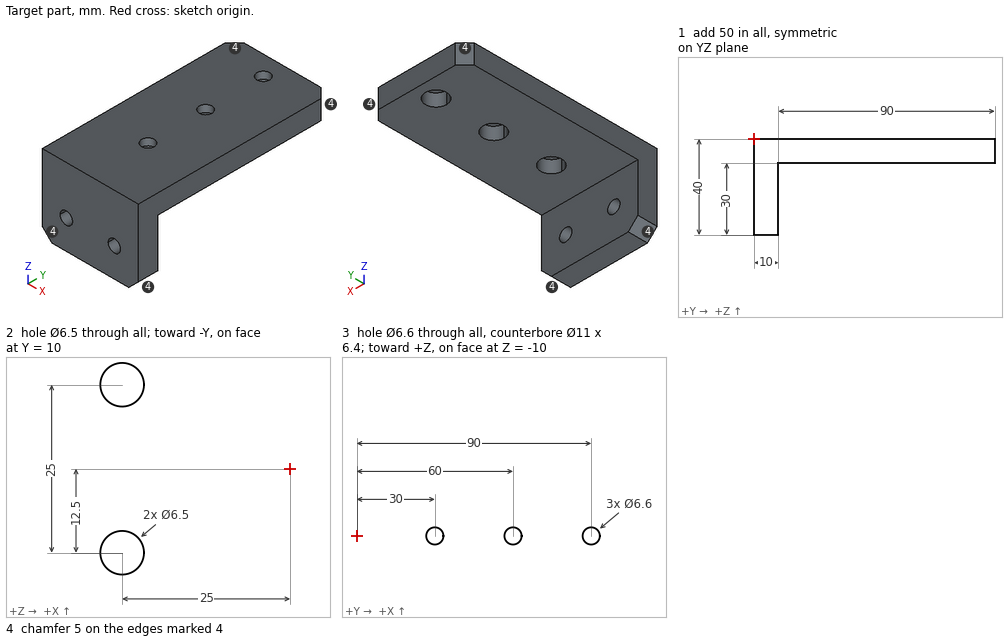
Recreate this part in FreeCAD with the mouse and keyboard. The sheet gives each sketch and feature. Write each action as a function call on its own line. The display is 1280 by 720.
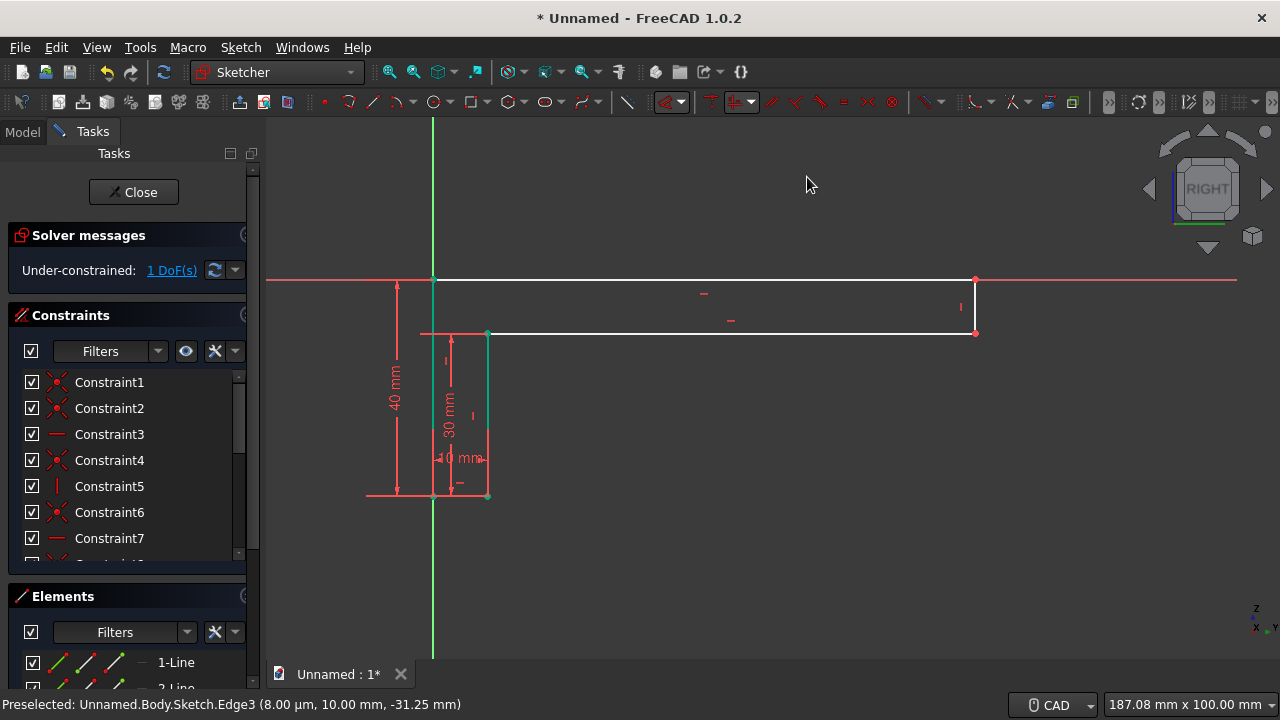
click(634, 334)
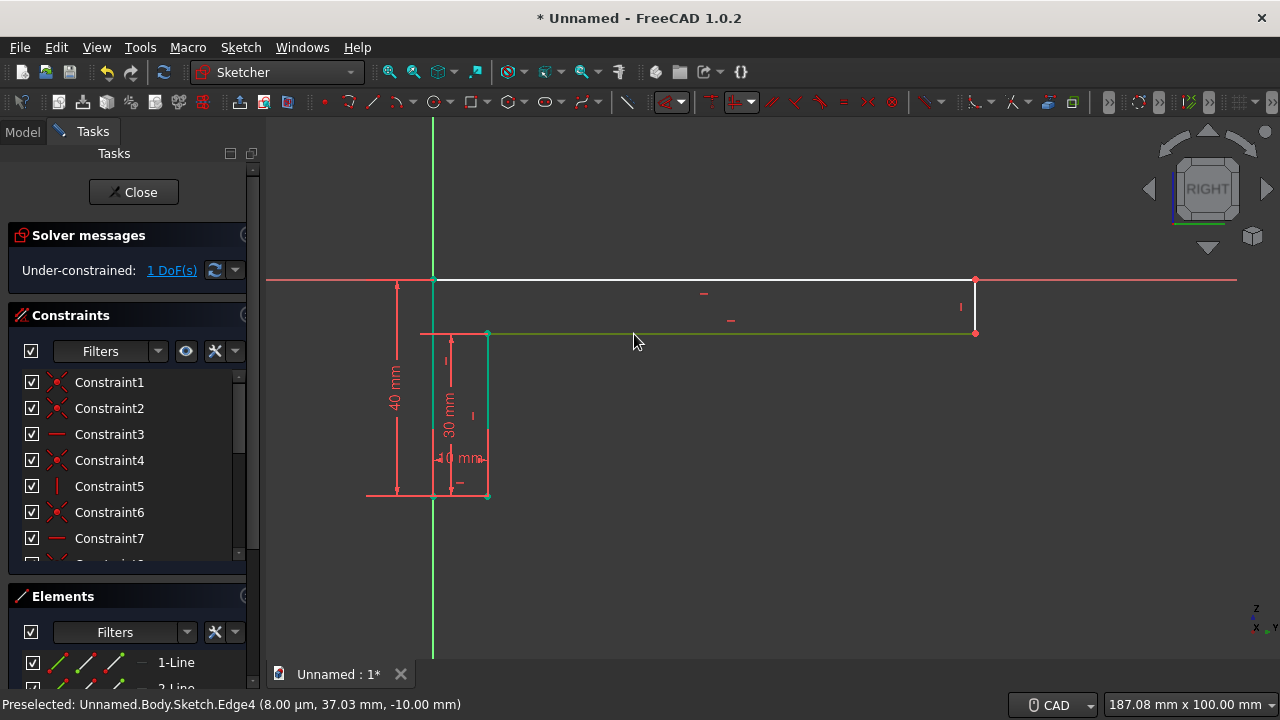
key(l)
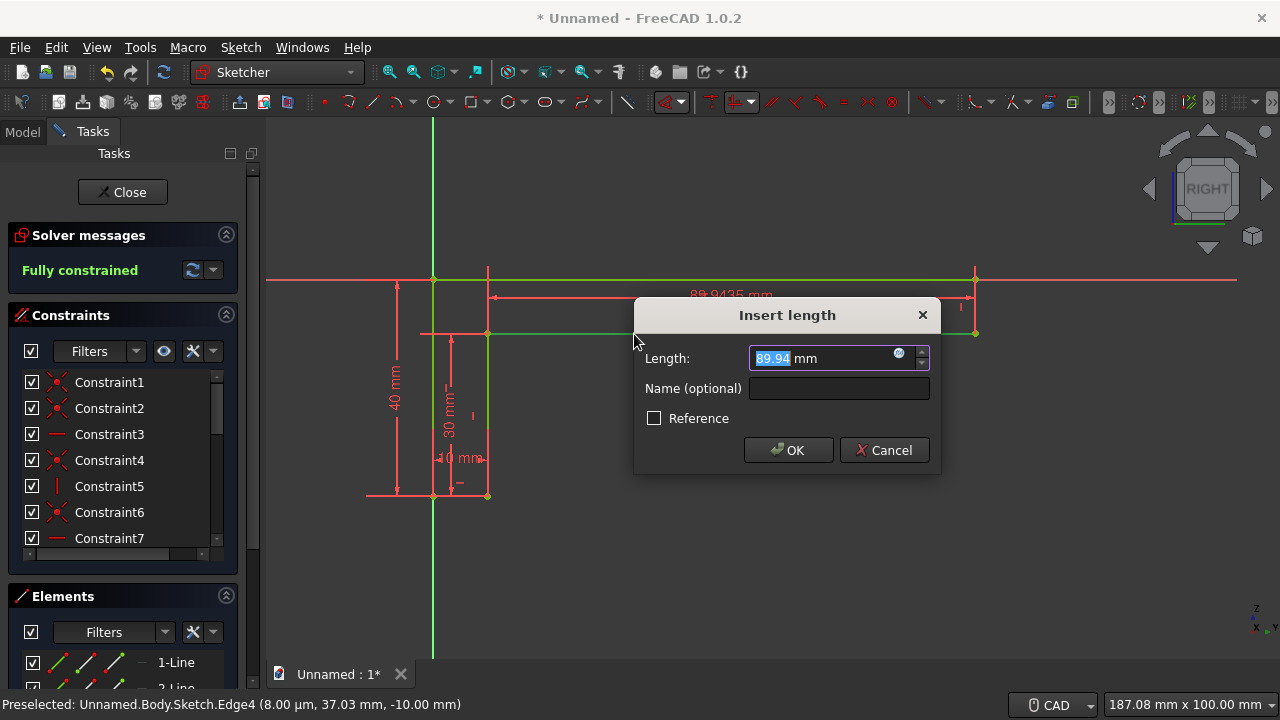
text(90)
key(Return)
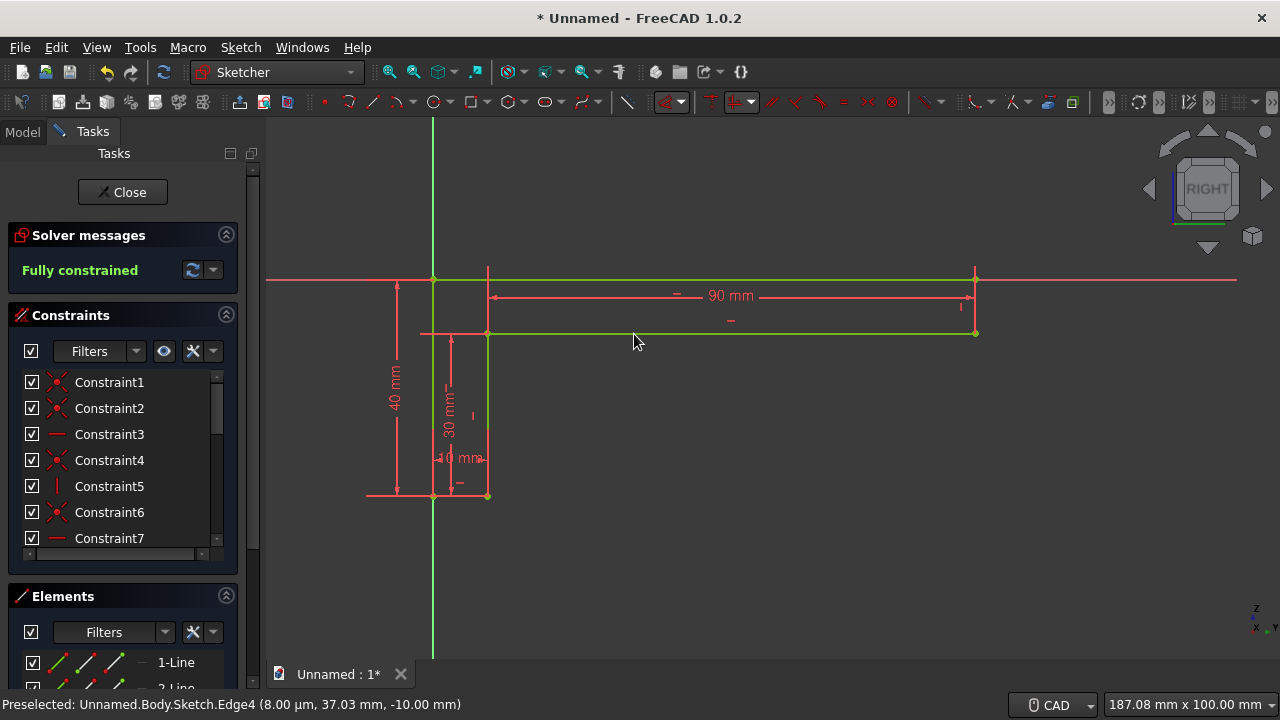
click(123, 192)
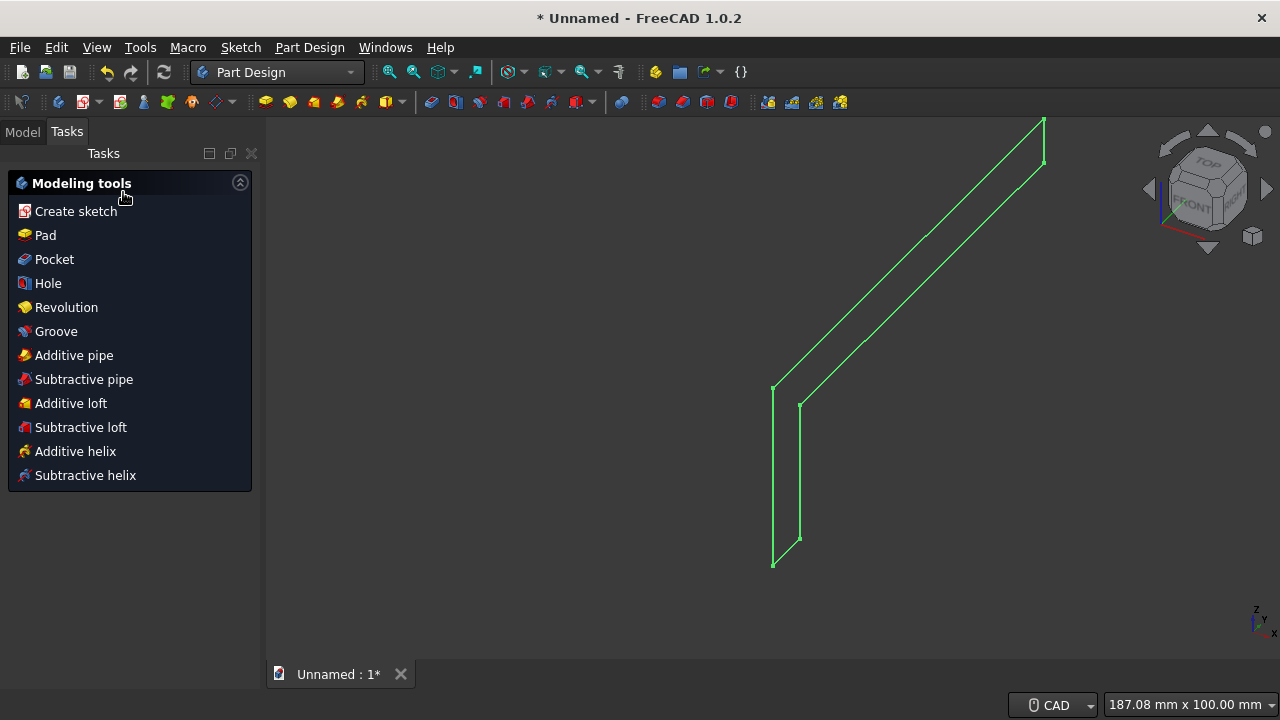
click(266, 102)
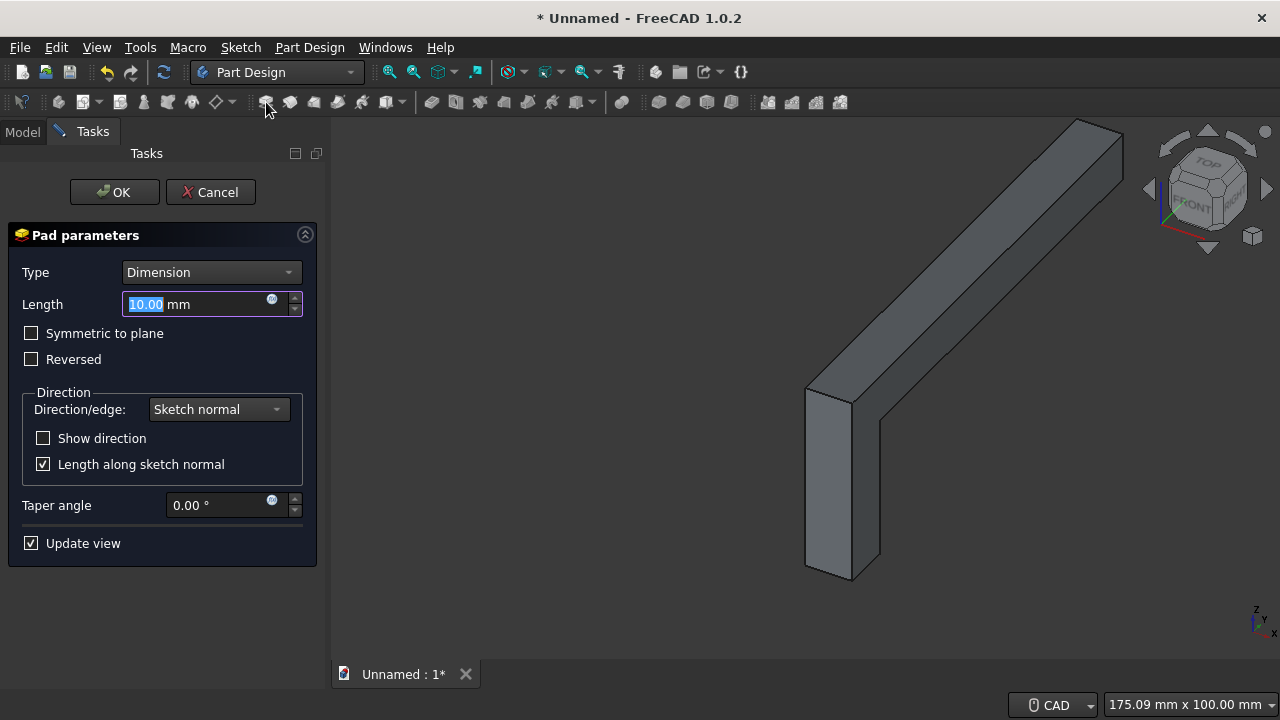
text(50)
key(Tab)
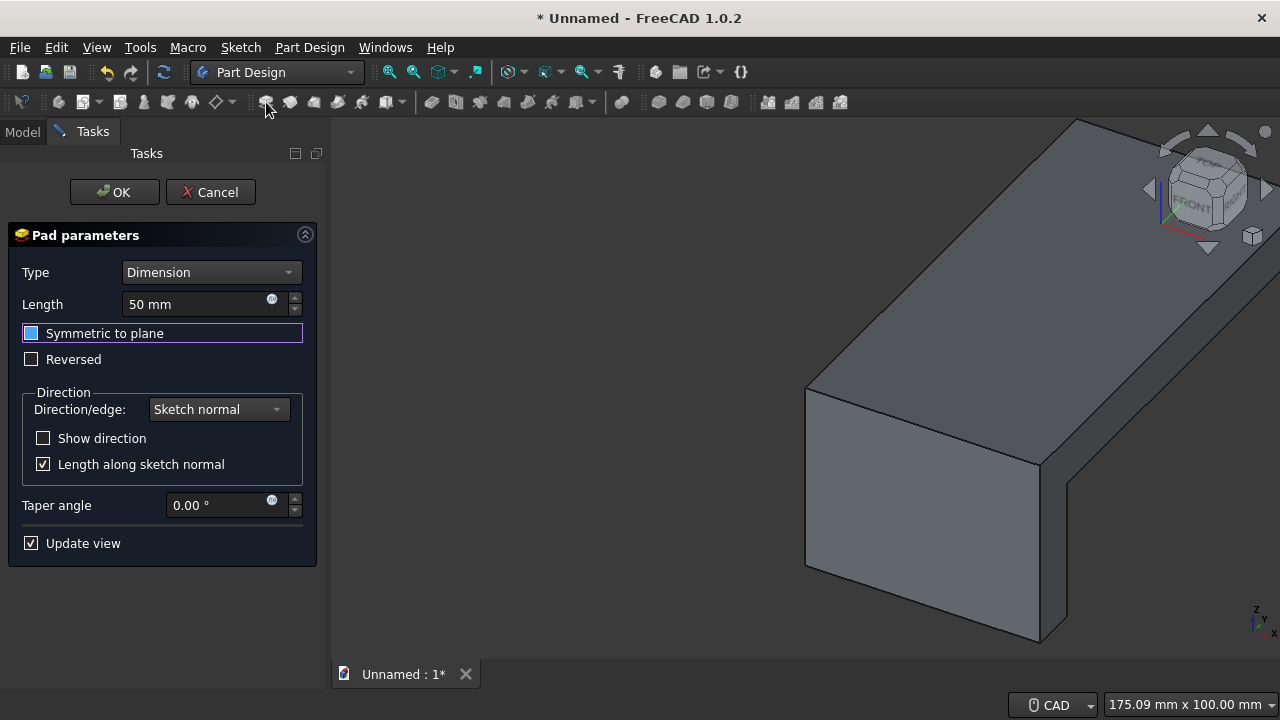
click(30, 333)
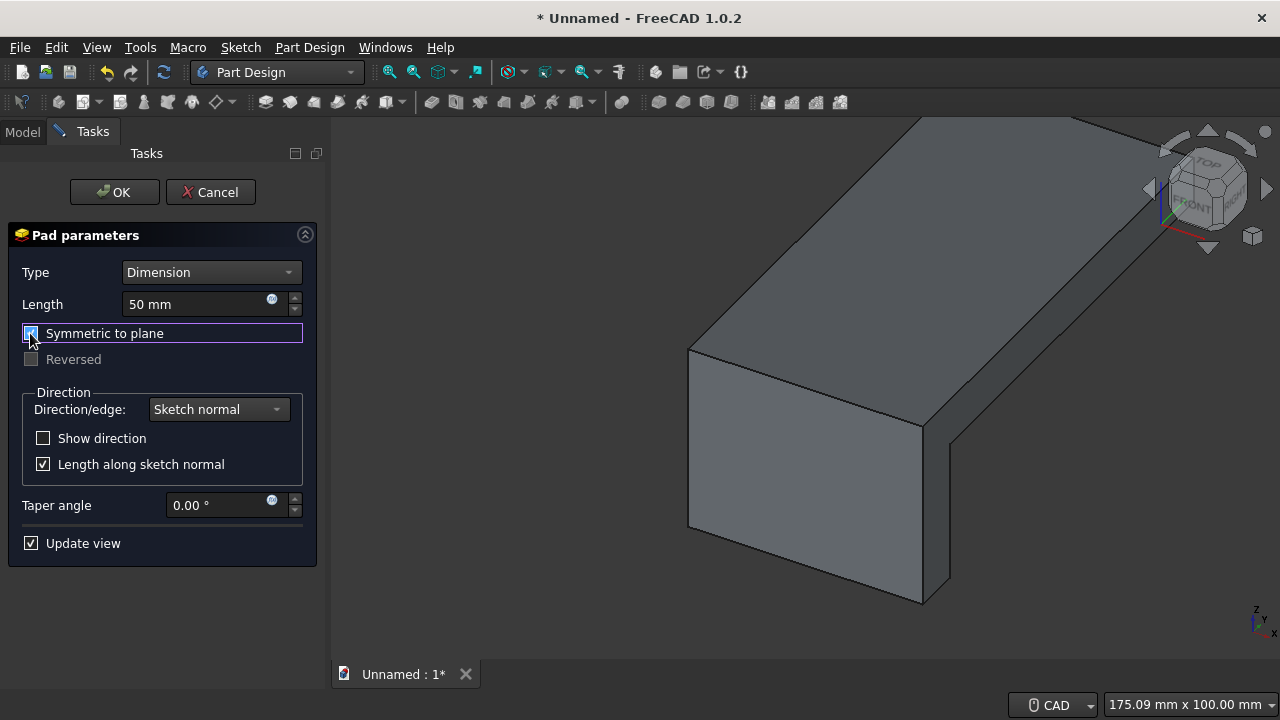
click(115, 192)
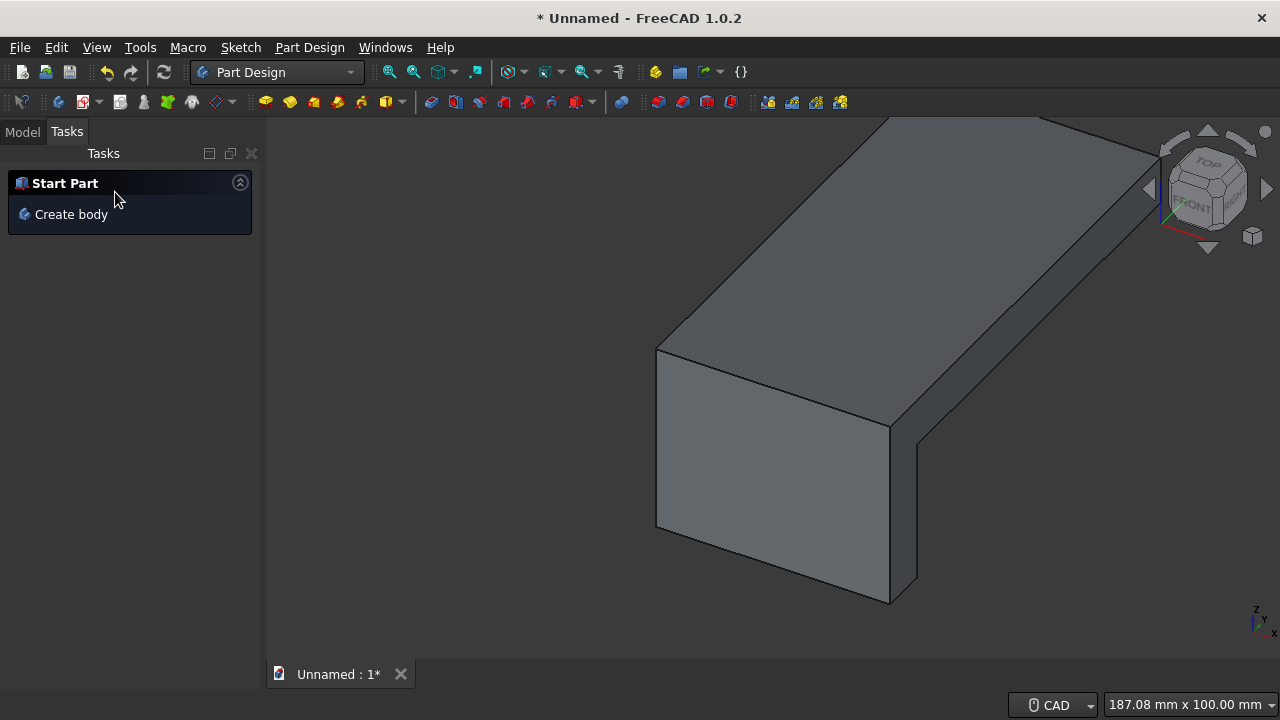
click(390, 72)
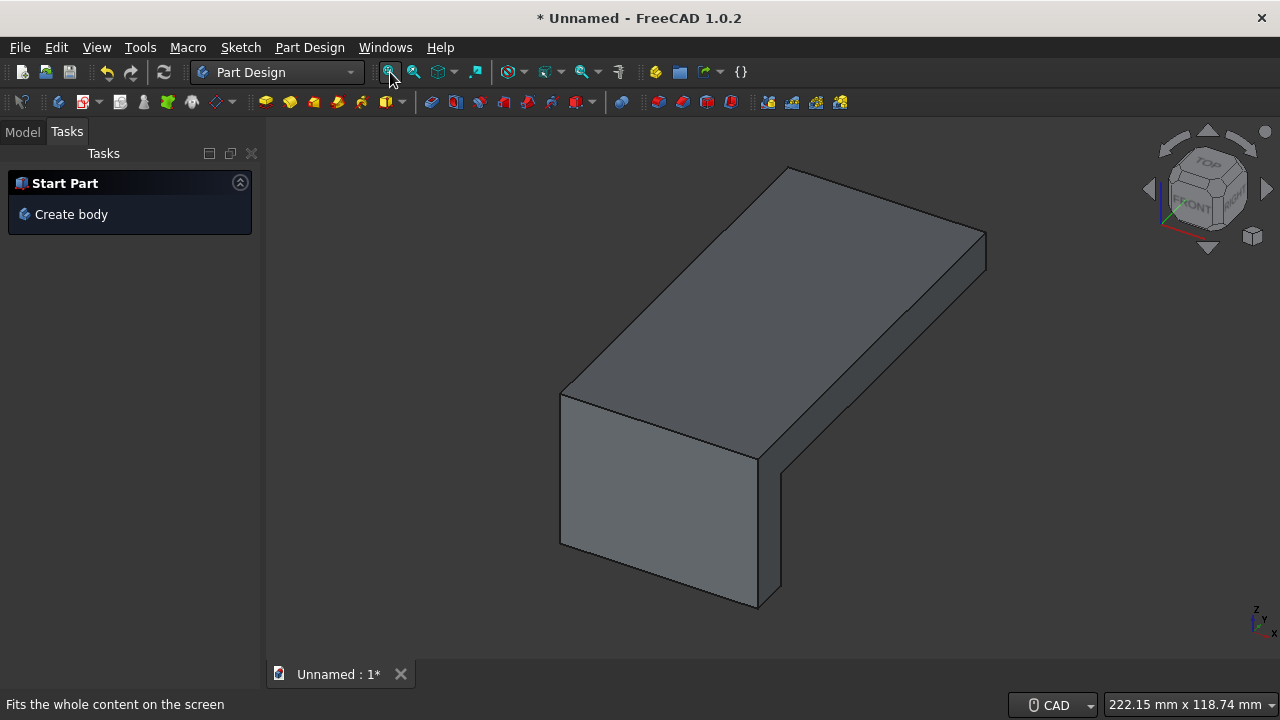
key(4)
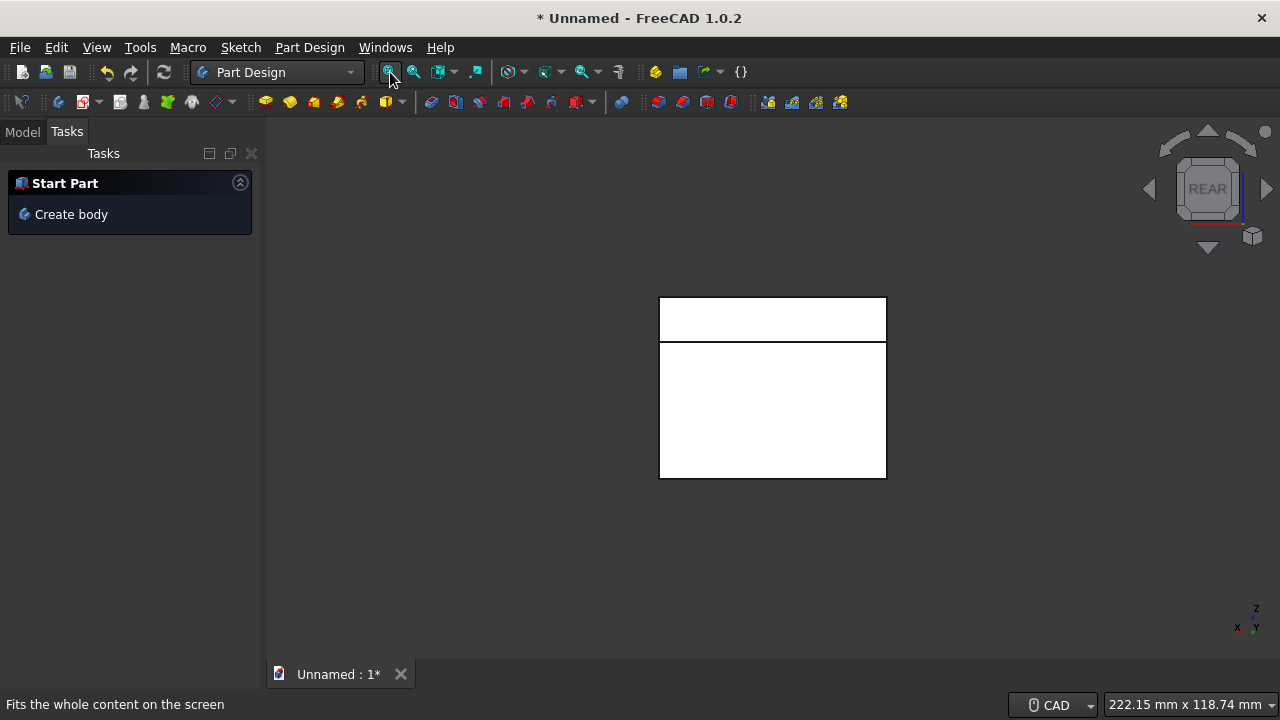
click(390, 72)